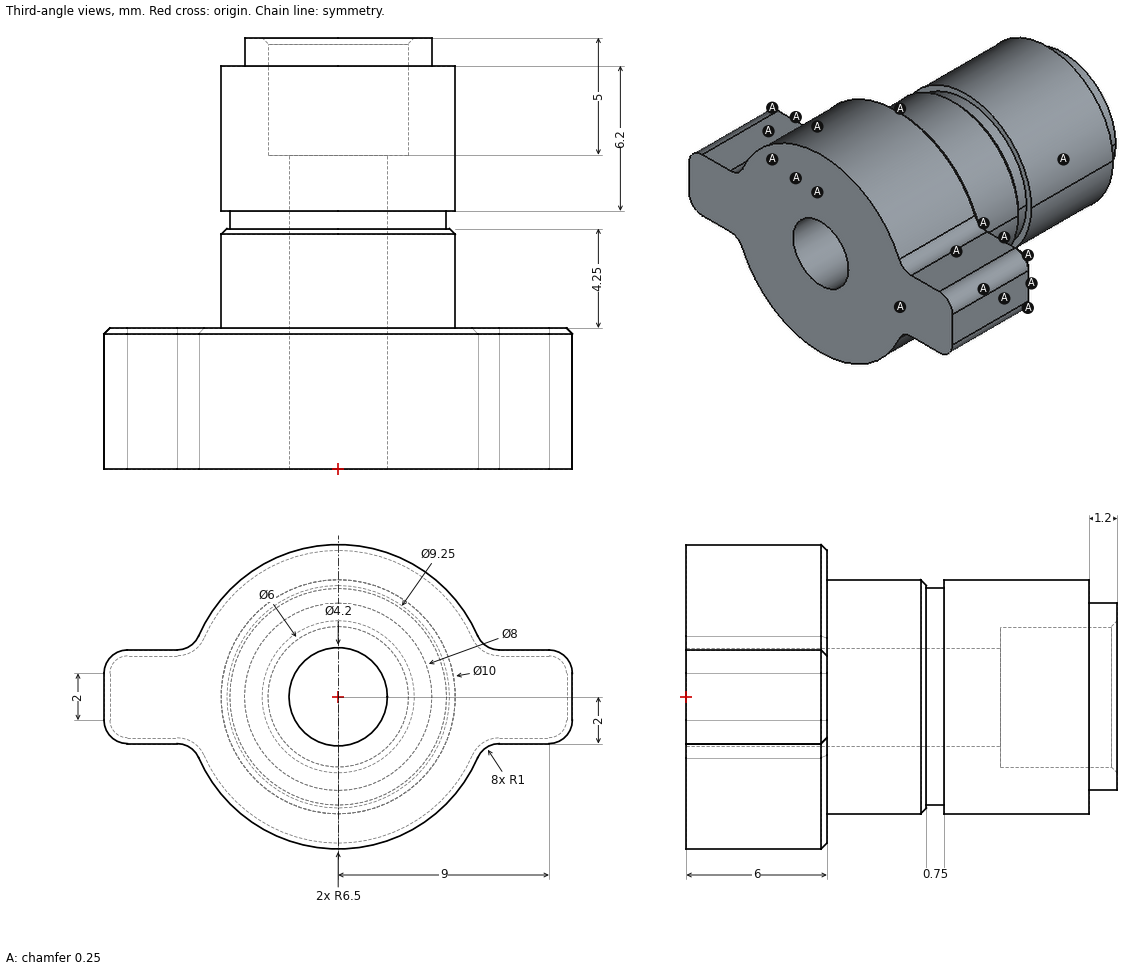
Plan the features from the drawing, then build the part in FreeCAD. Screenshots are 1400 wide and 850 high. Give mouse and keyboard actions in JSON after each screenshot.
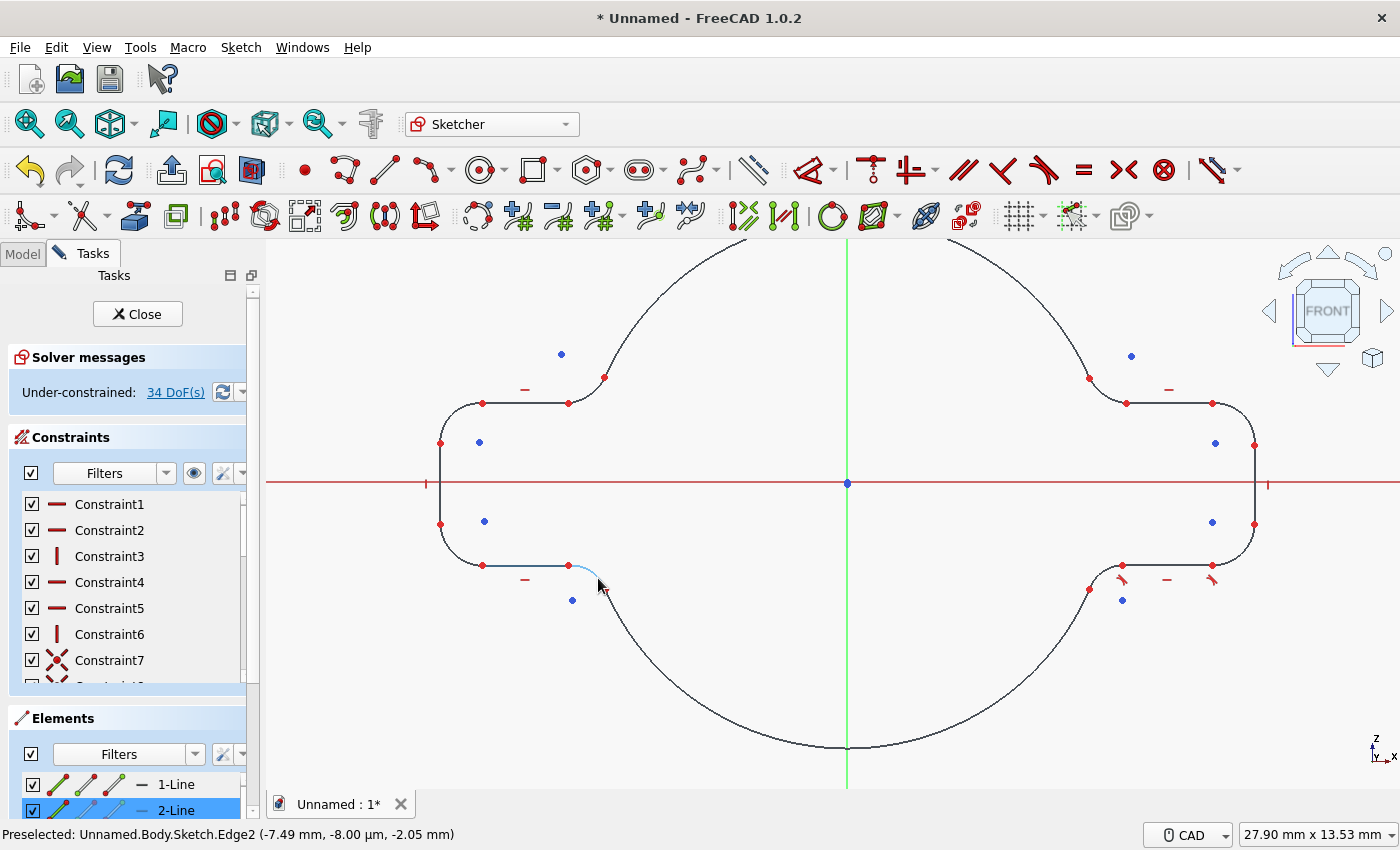
{"action": "left_click", "coordinate": [598, 577]}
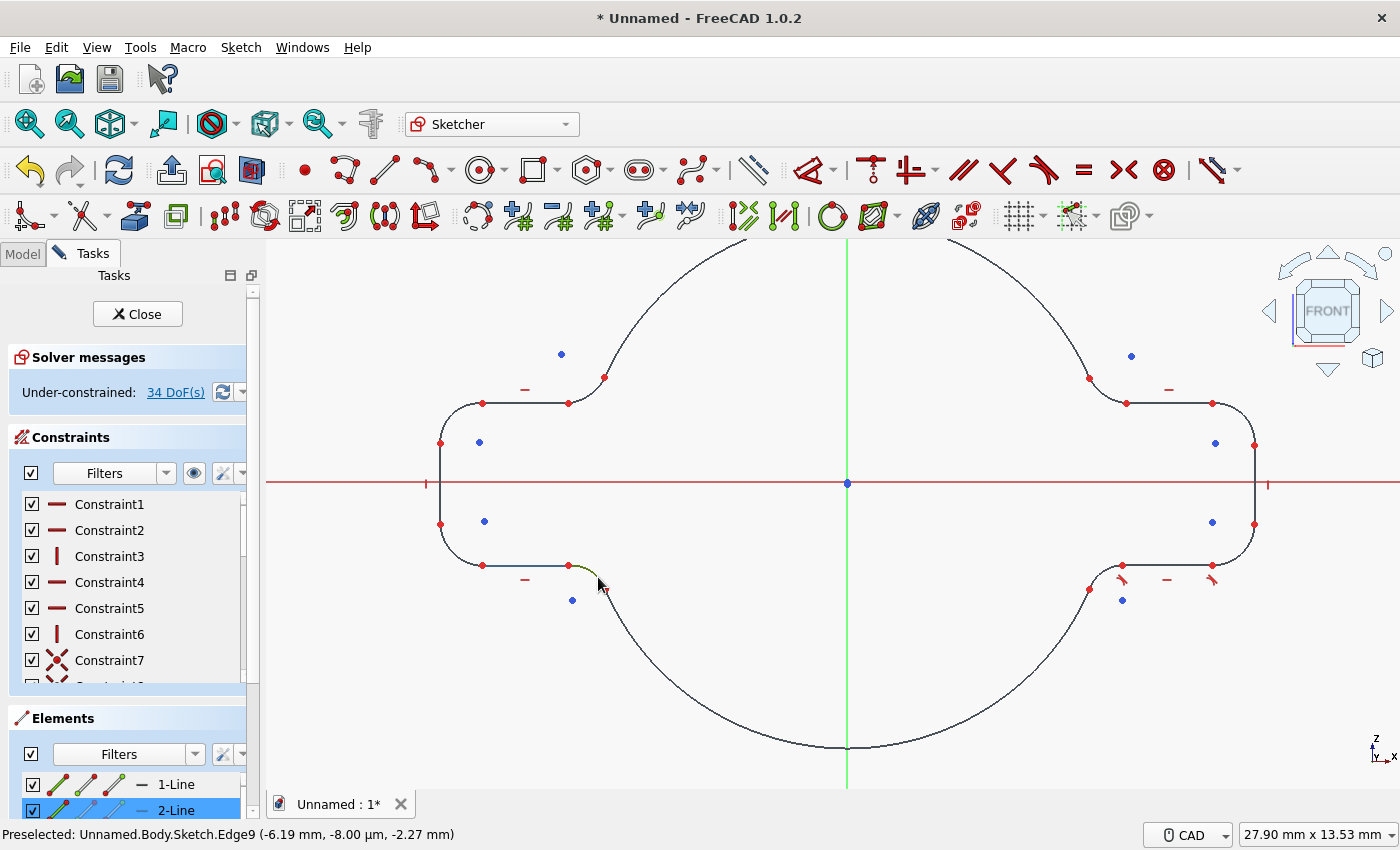
{"action": "left_click", "coordinate": [1044, 170]}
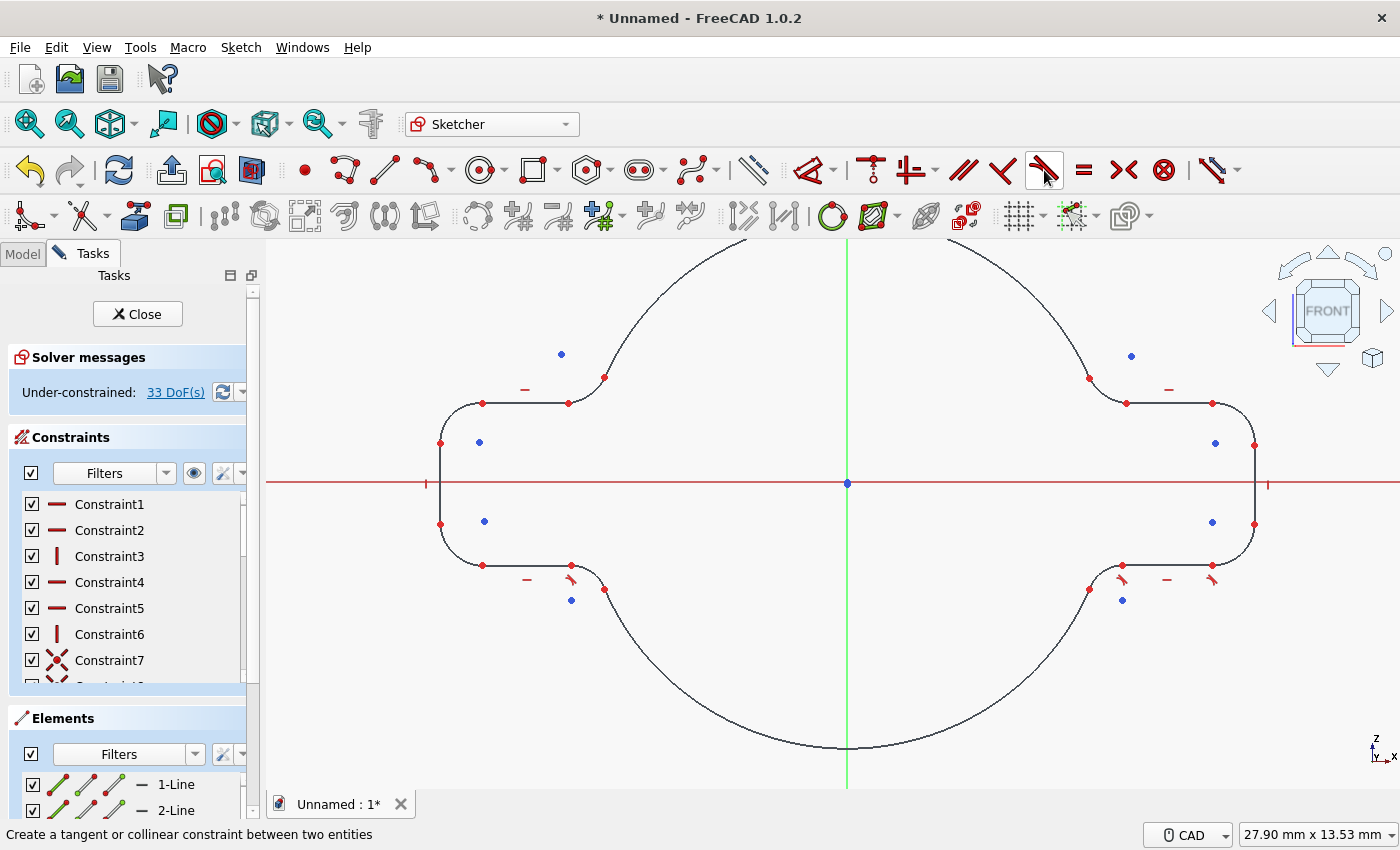
{"action": "left_click", "coordinate": [545, 566]}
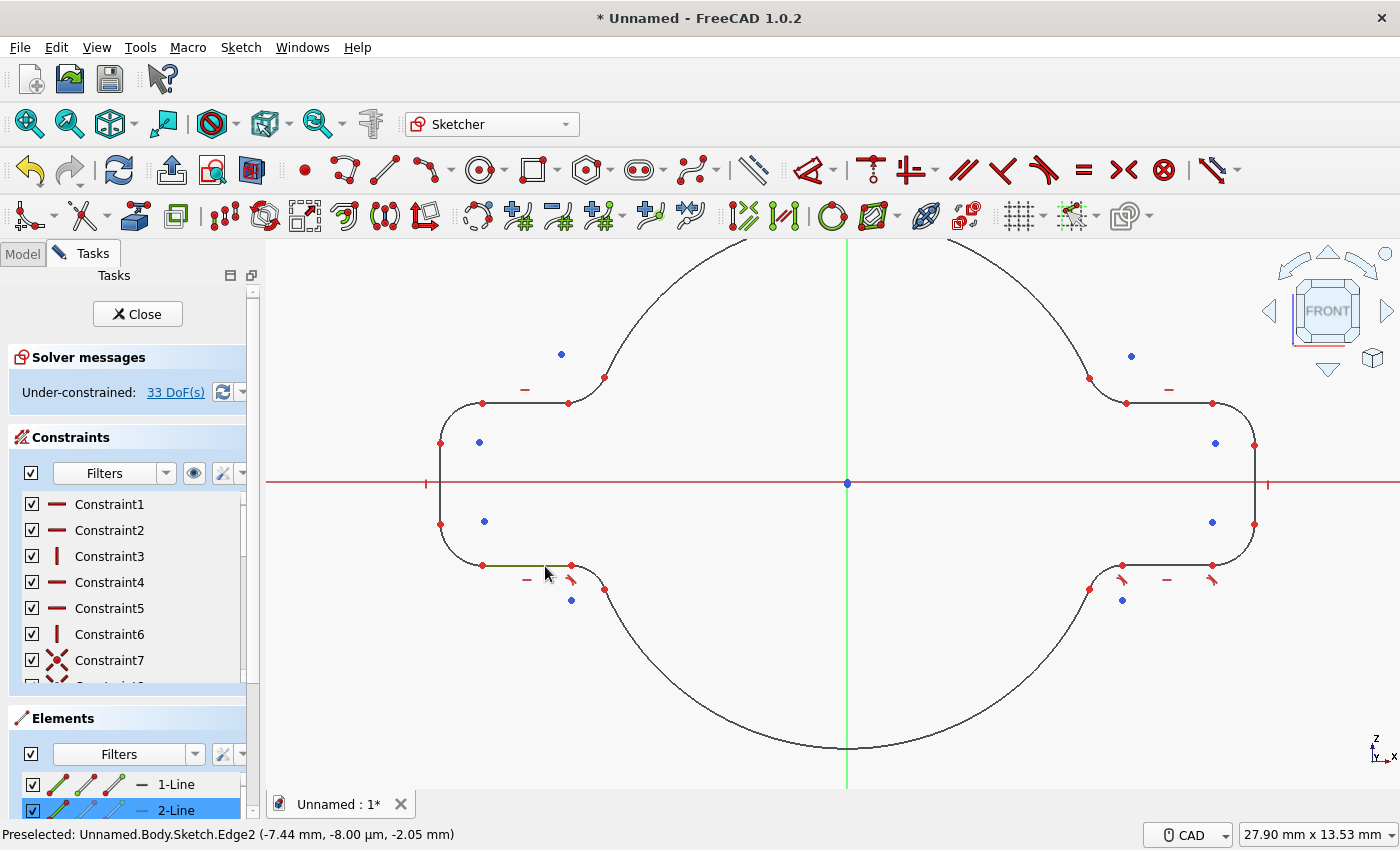
{"action": "left_click", "coordinate": [446, 543]}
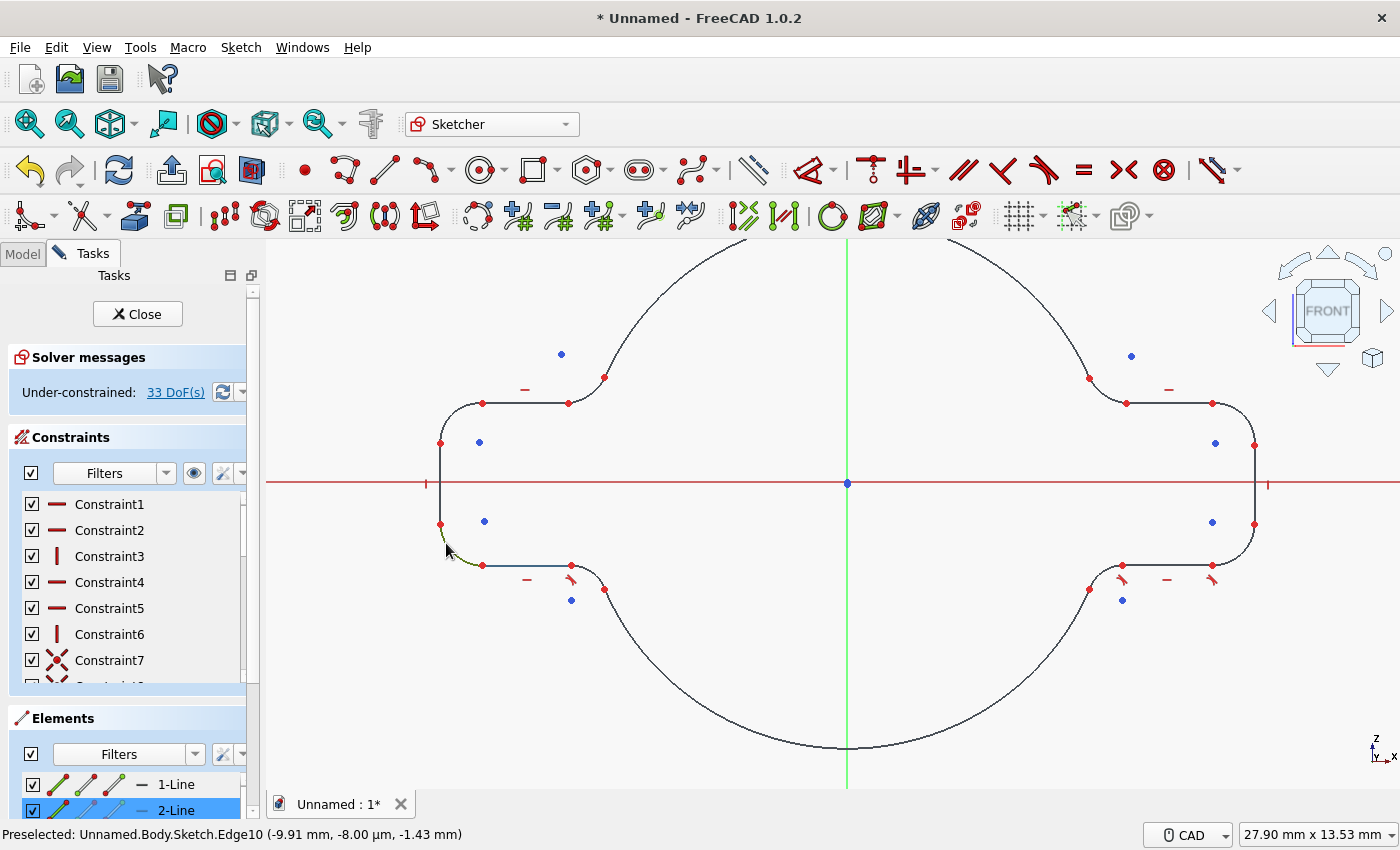
{"action": "left_click", "coordinate": [1044, 170]}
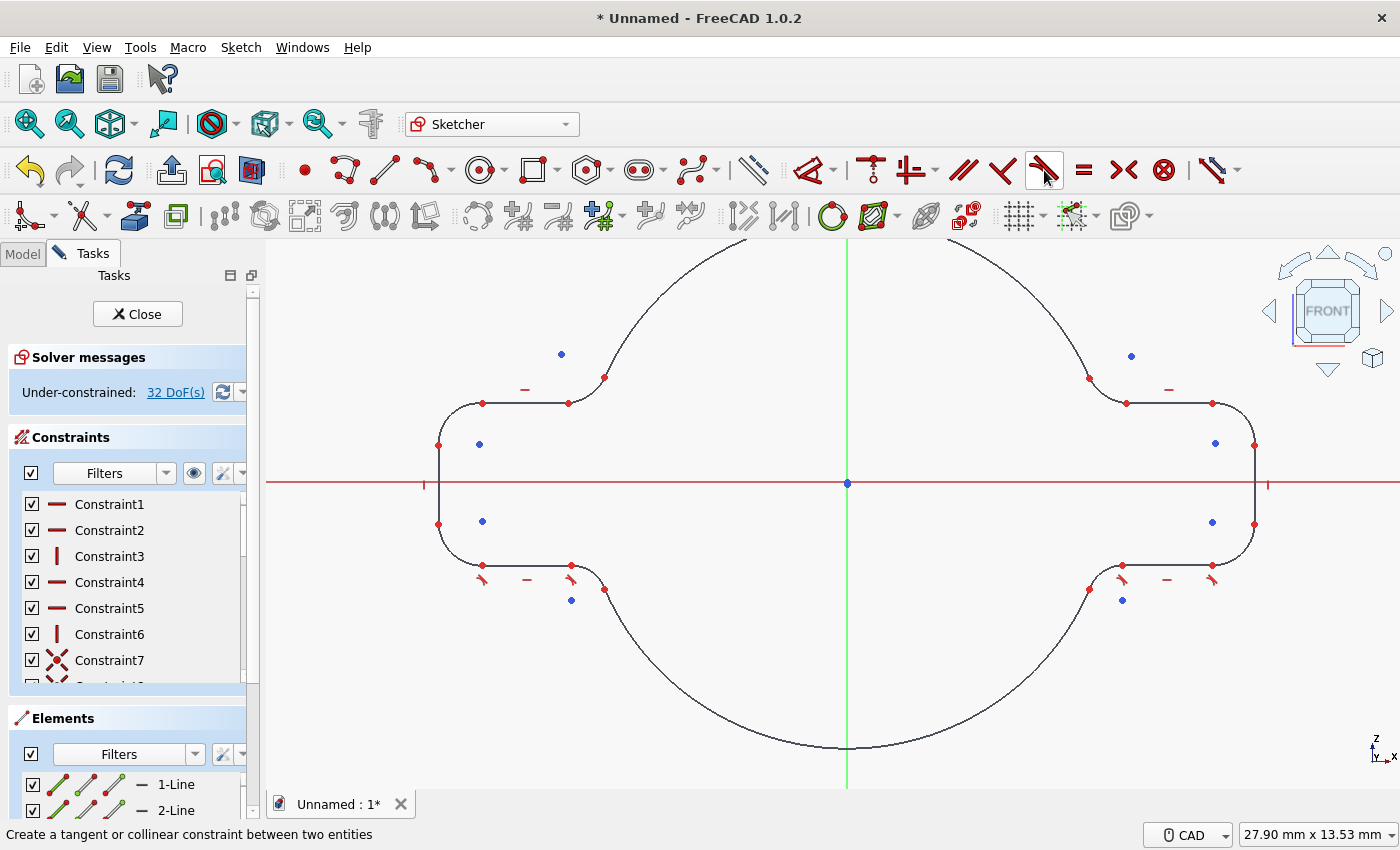
{"action": "left_click", "coordinate": [439, 500]}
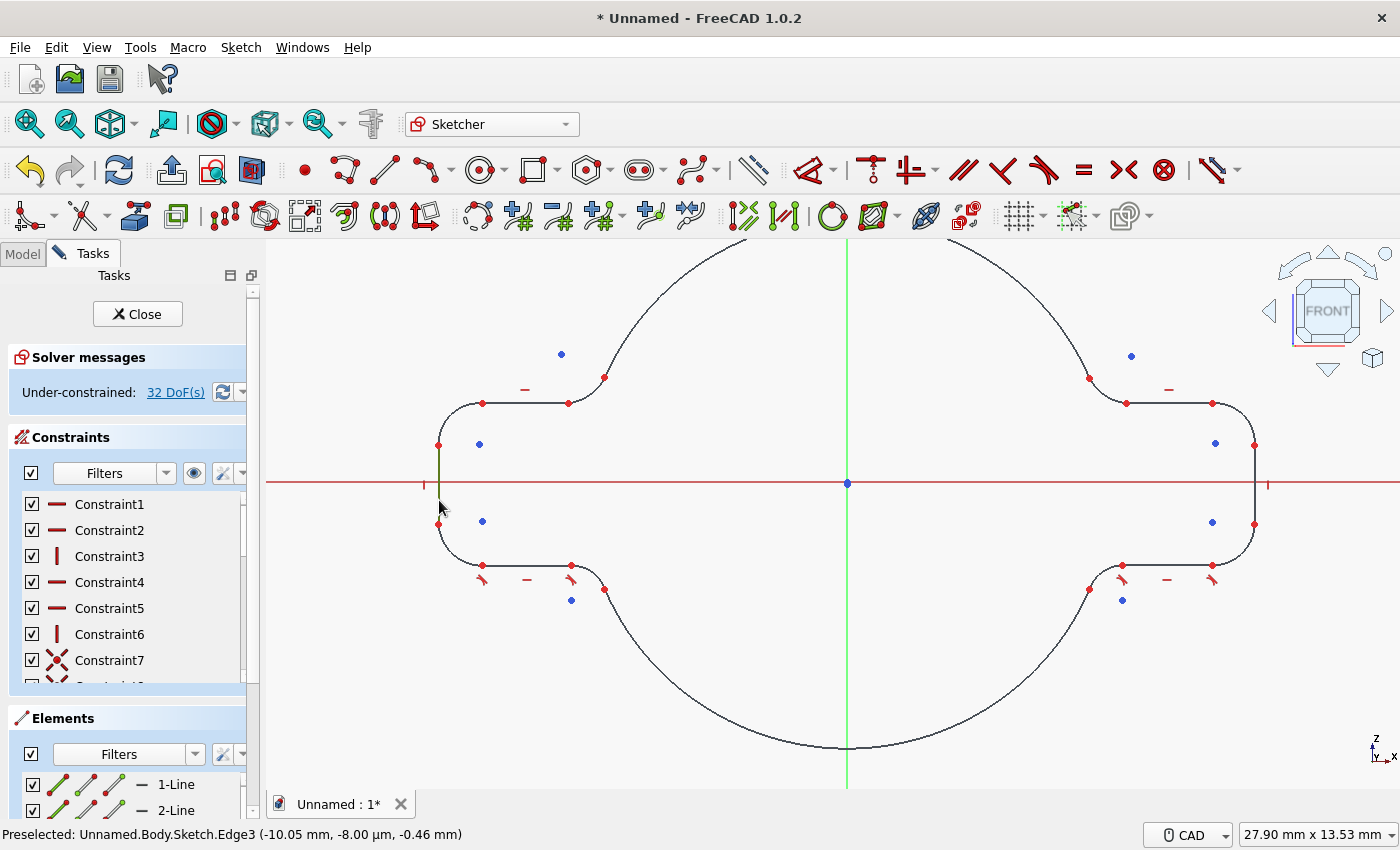
{"action": "left_click", "coordinate": [444, 543]}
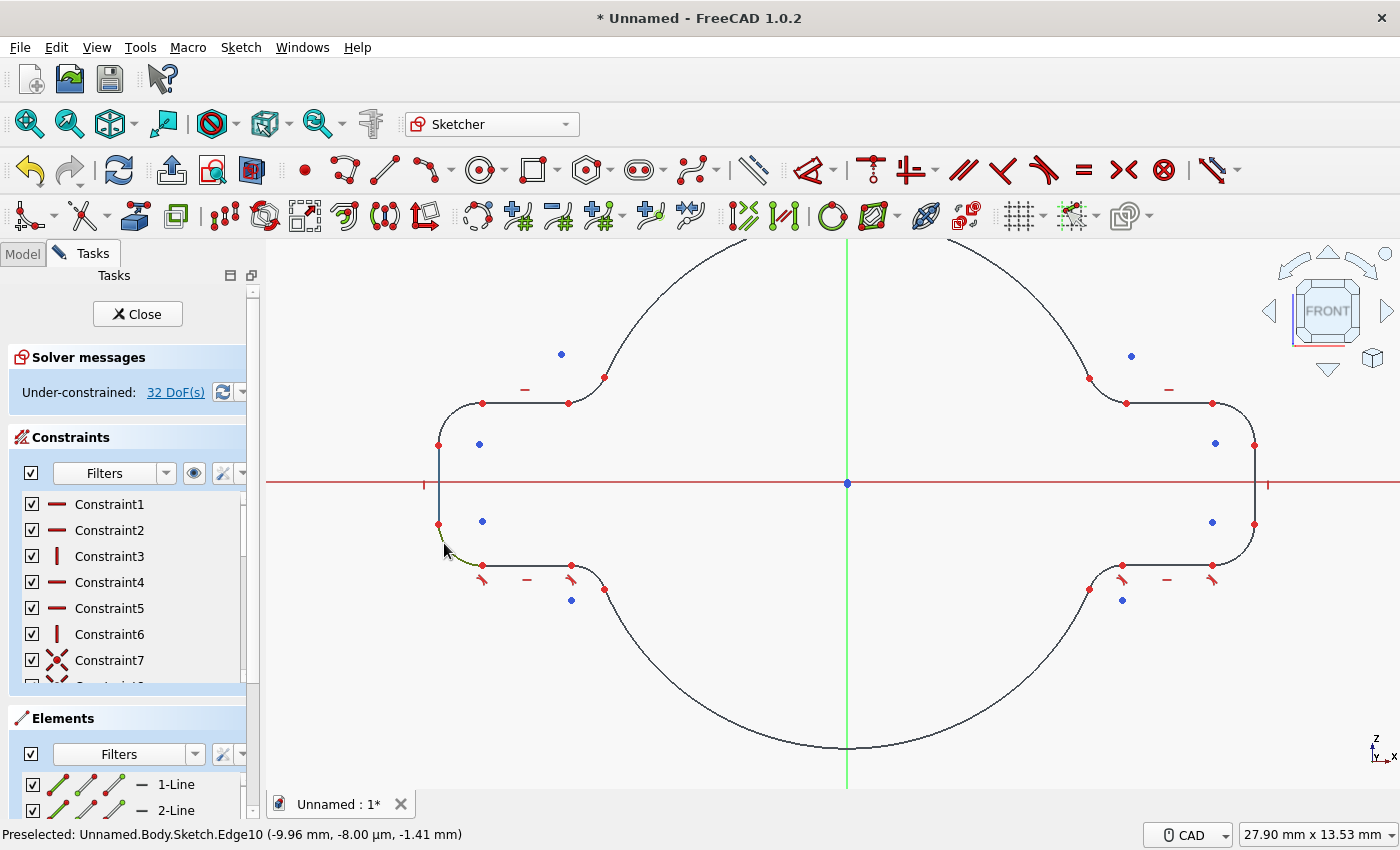
{"action": "left_click", "coordinate": [1044, 170]}